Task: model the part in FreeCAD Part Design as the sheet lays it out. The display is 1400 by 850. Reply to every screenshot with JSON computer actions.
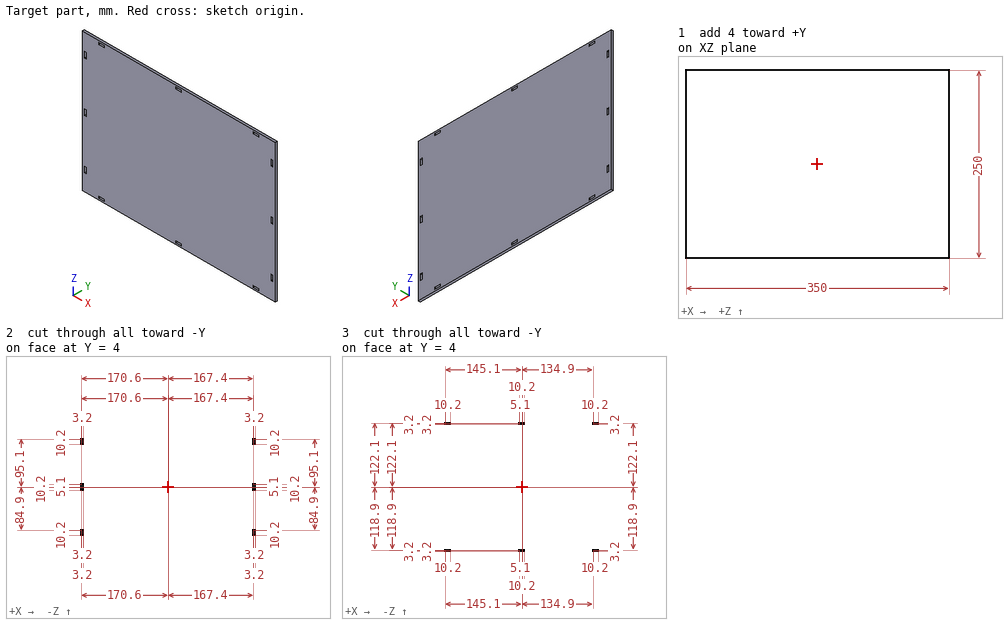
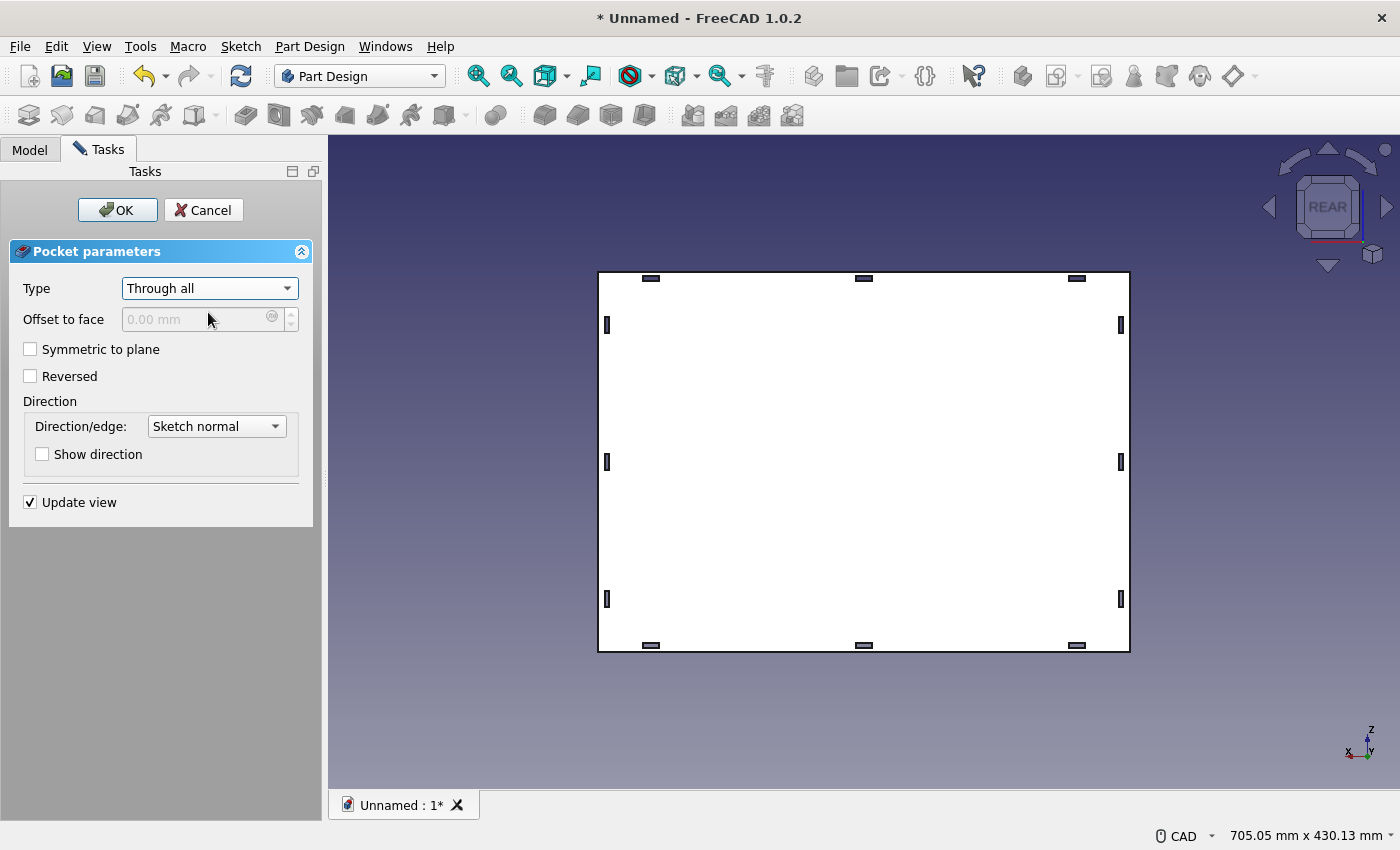
{"action": "left_click", "coordinate": [118, 210]}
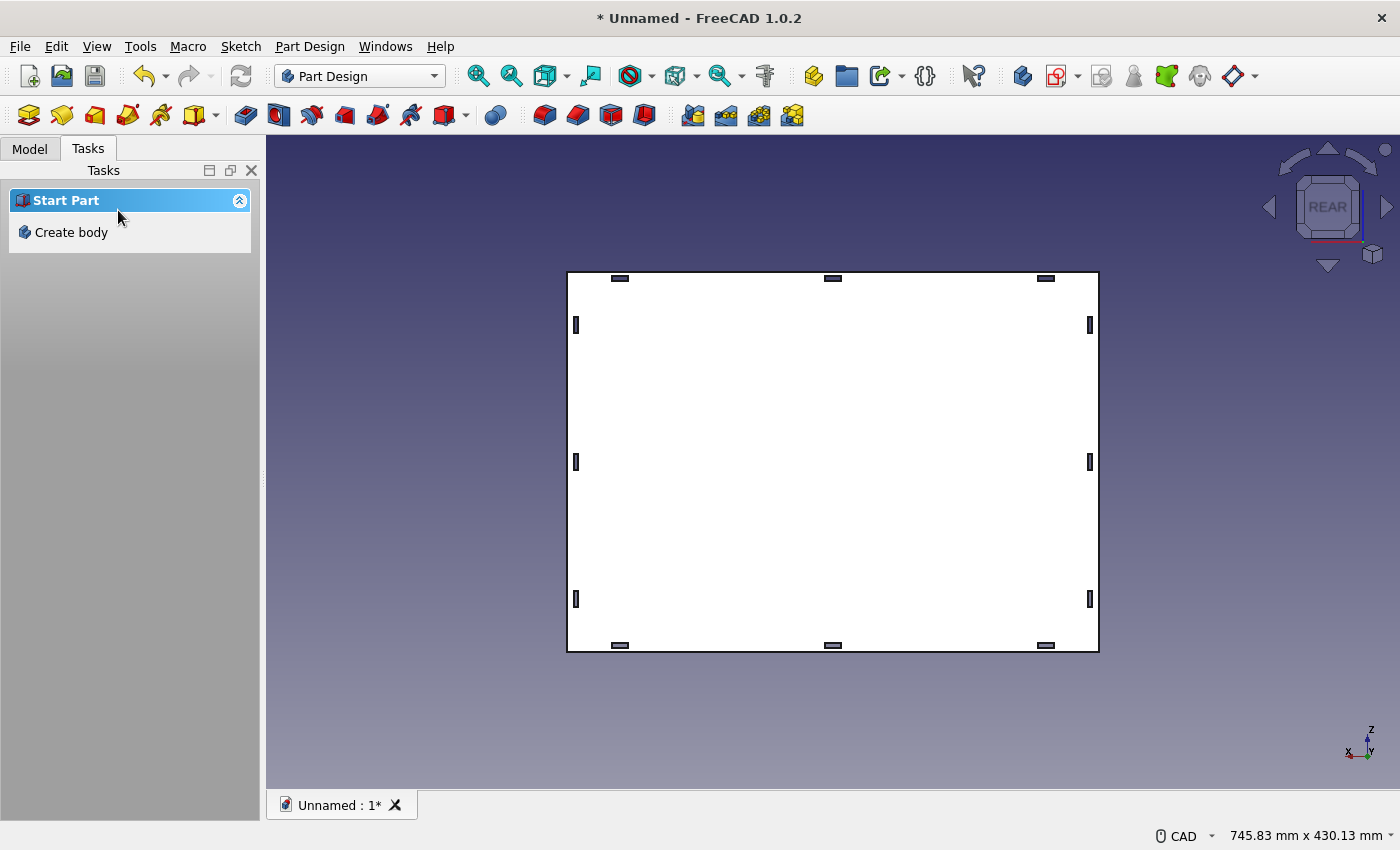
{"action": "key", "text": "0"}